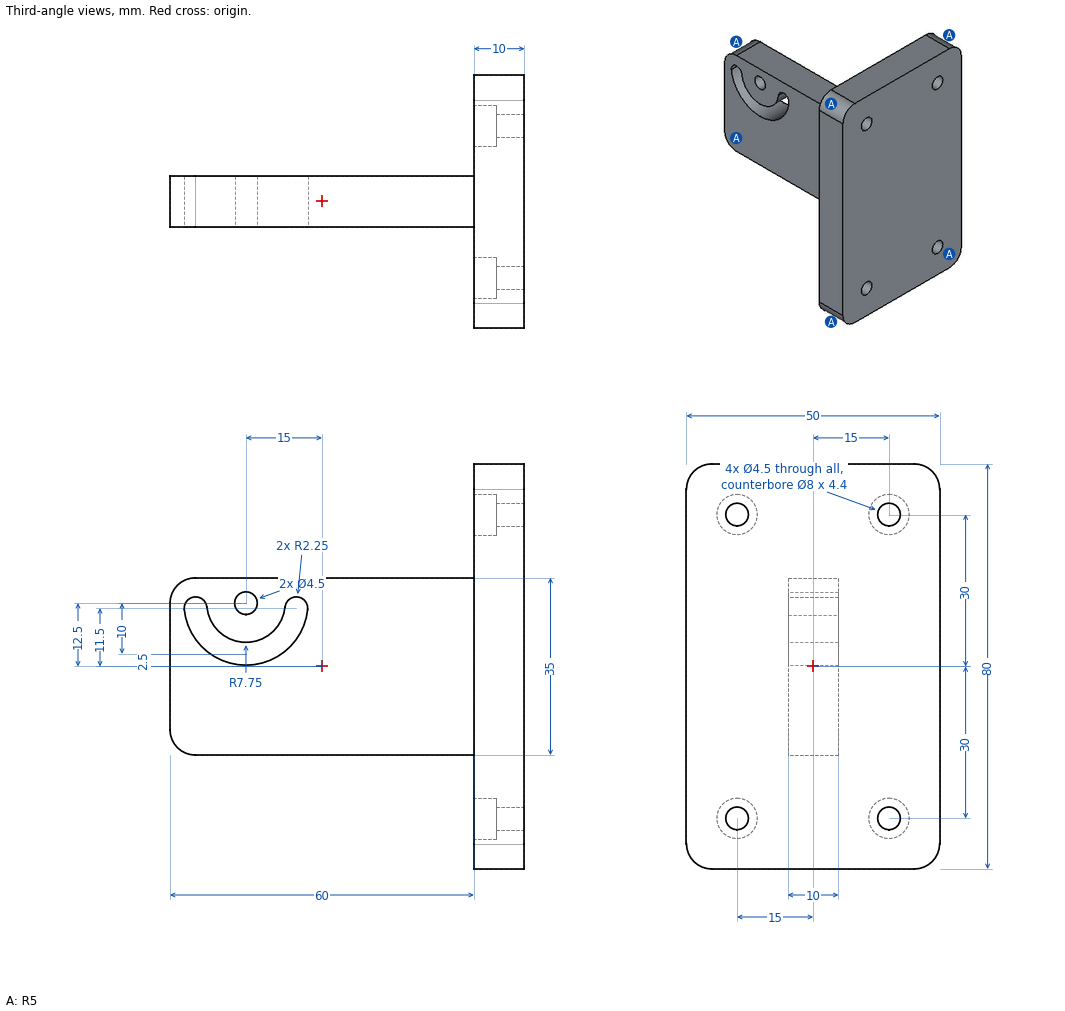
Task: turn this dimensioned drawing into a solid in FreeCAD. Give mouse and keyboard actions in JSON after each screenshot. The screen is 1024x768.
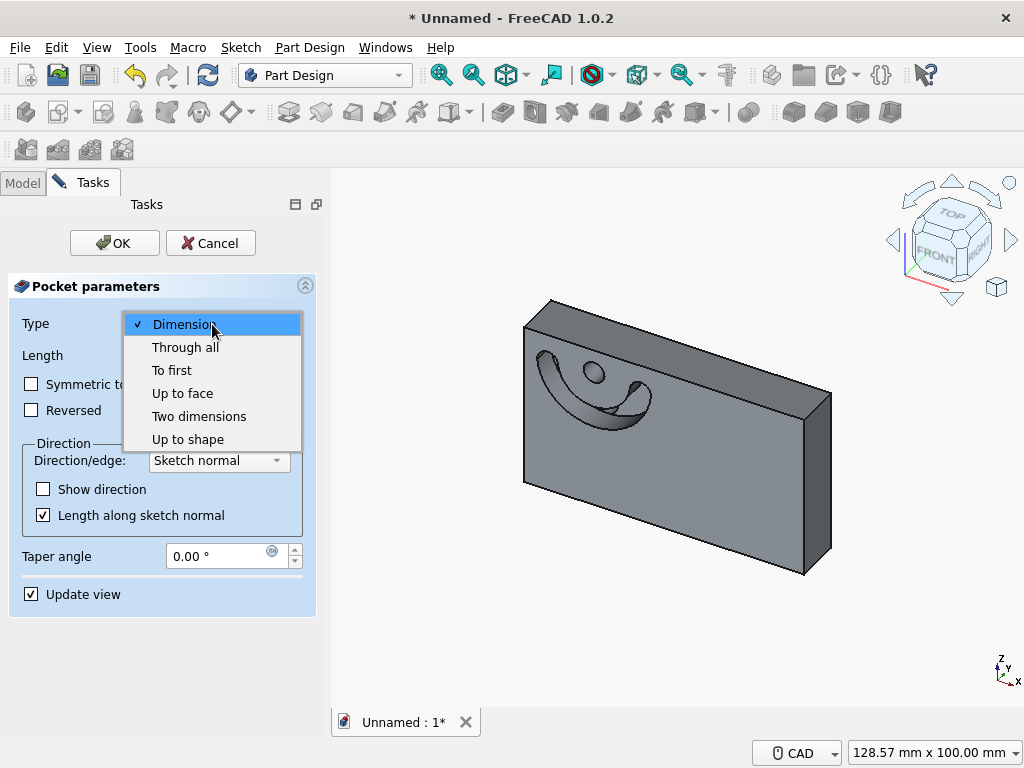
{"action": "left_click", "coordinate": [212, 348]}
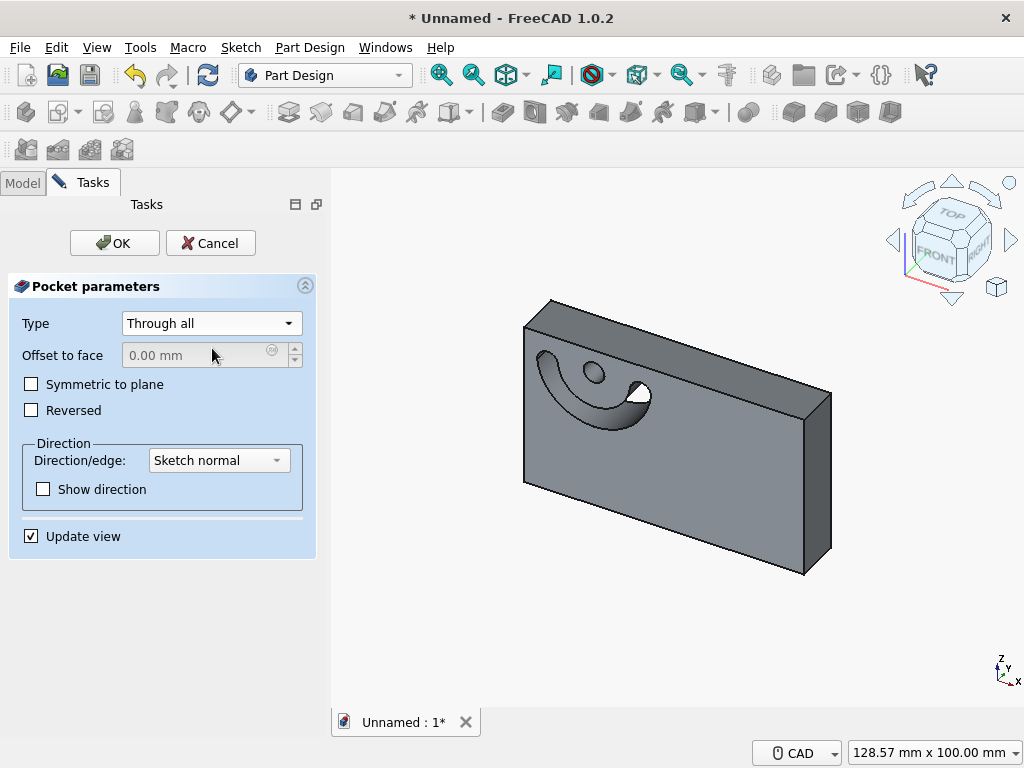
{"action": "left_click", "coordinate": [115, 243]}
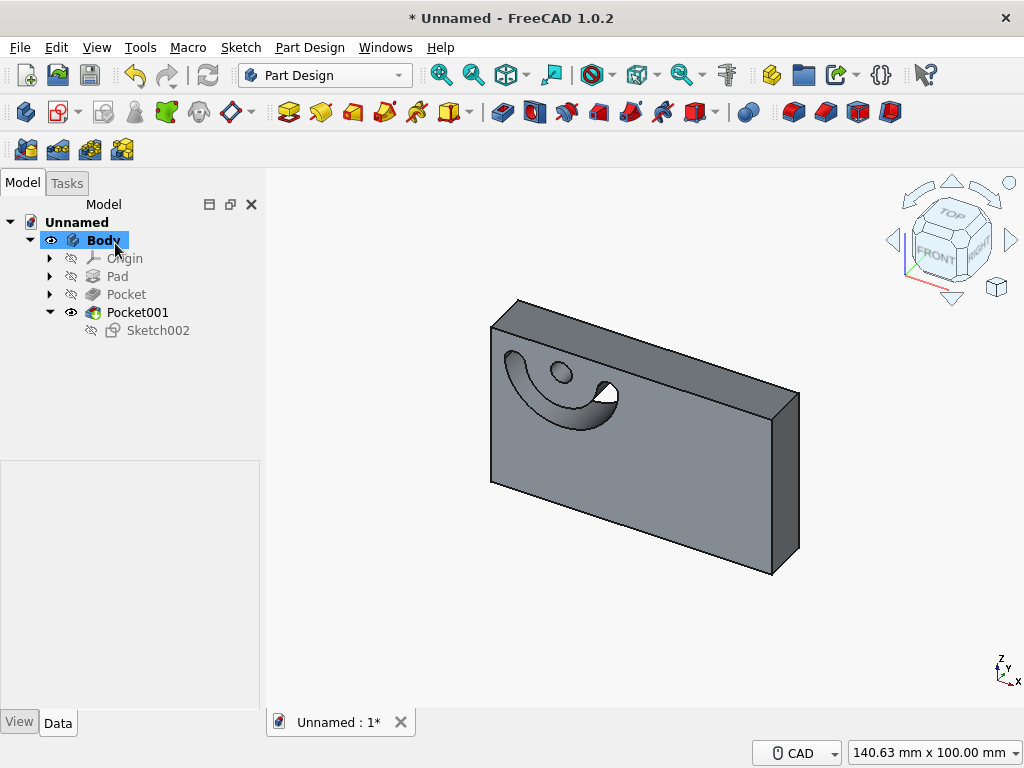
{"action": "left_click", "coordinate": [785, 439]}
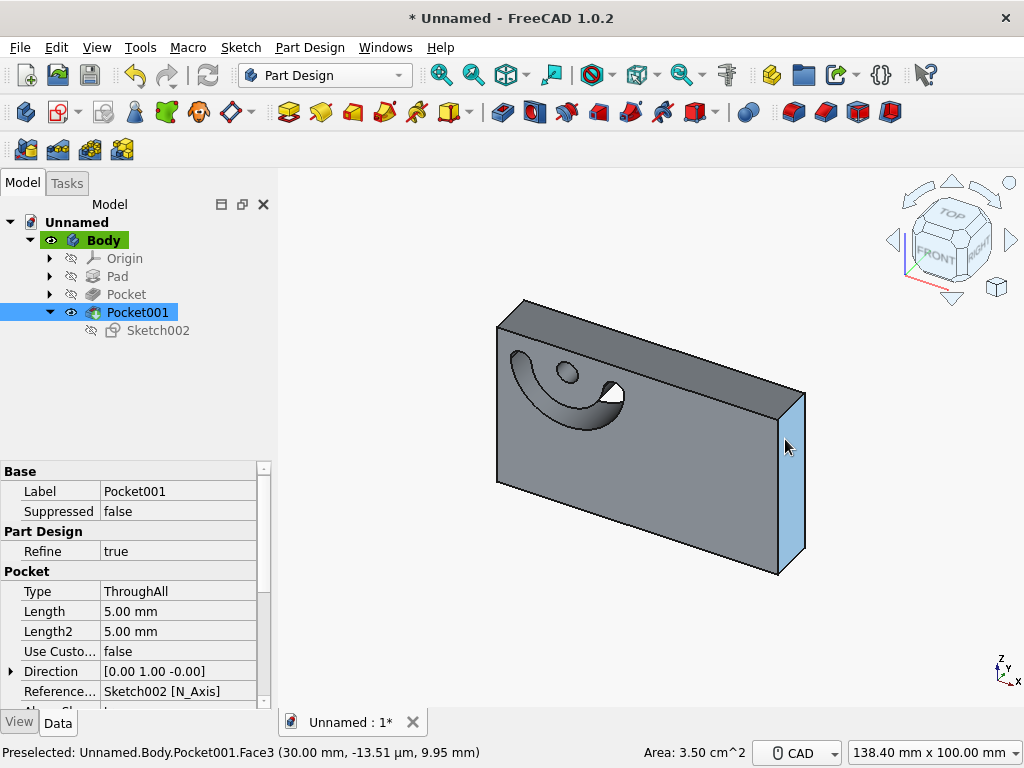
{"action": "left_click", "coordinate": [58, 112]}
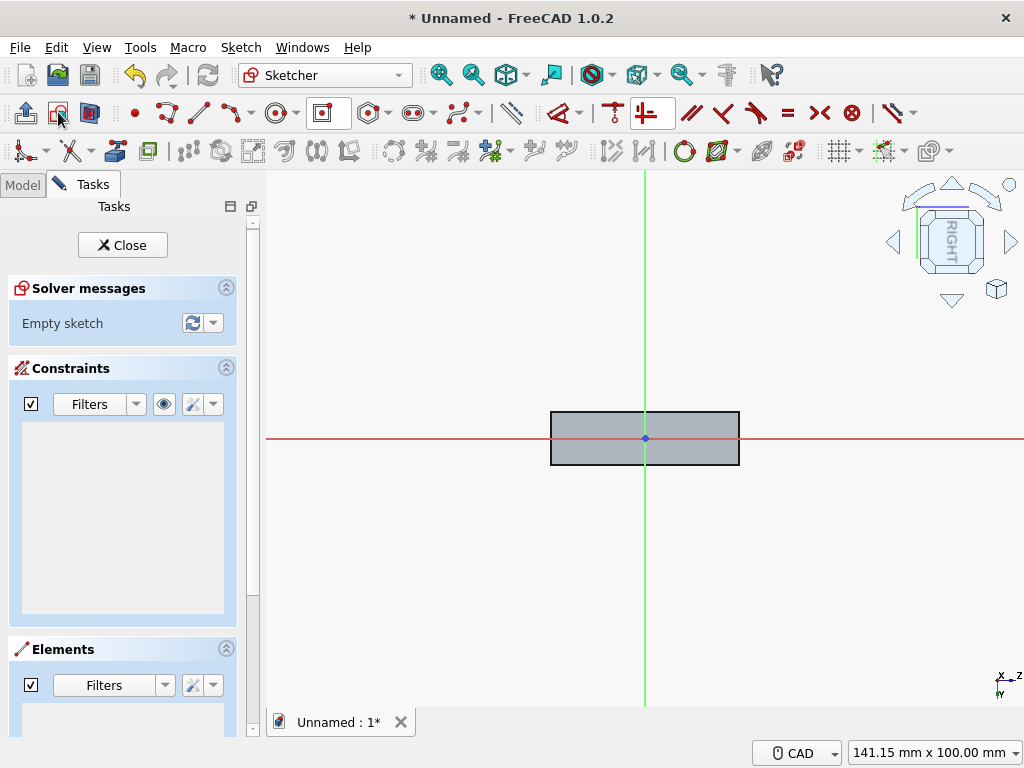
{"action": "scroll", "coordinate": [294, 439], "scroll_direction": "down", "scroll_amount": 1}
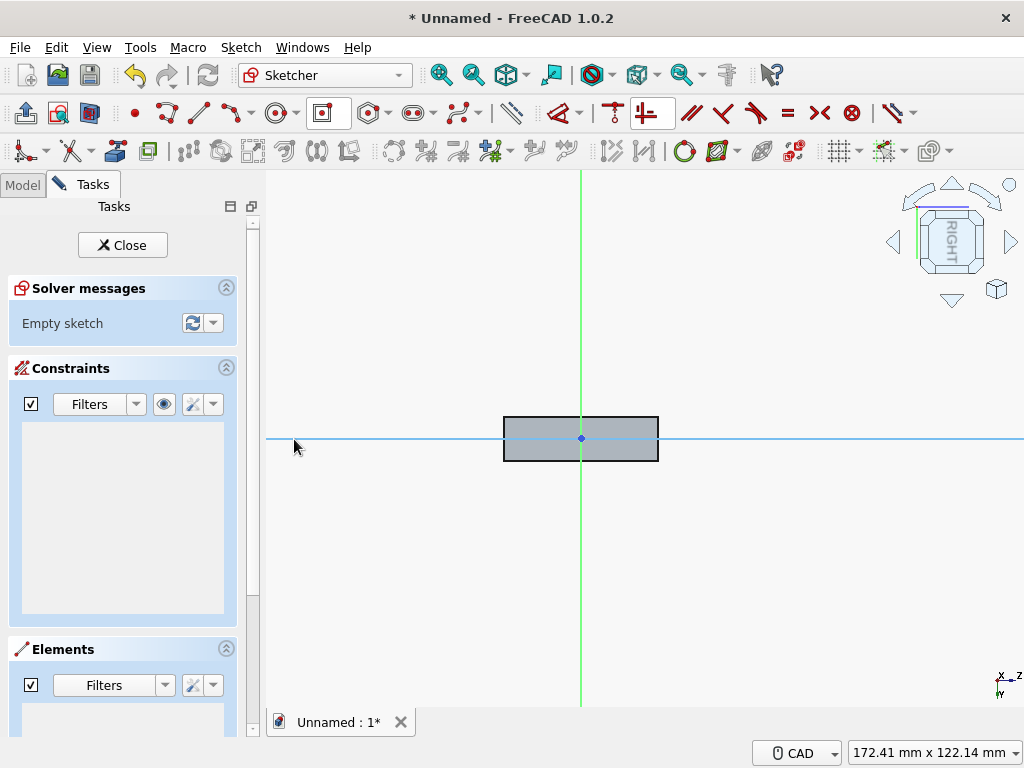
{"action": "left_click", "coordinate": [322, 114]}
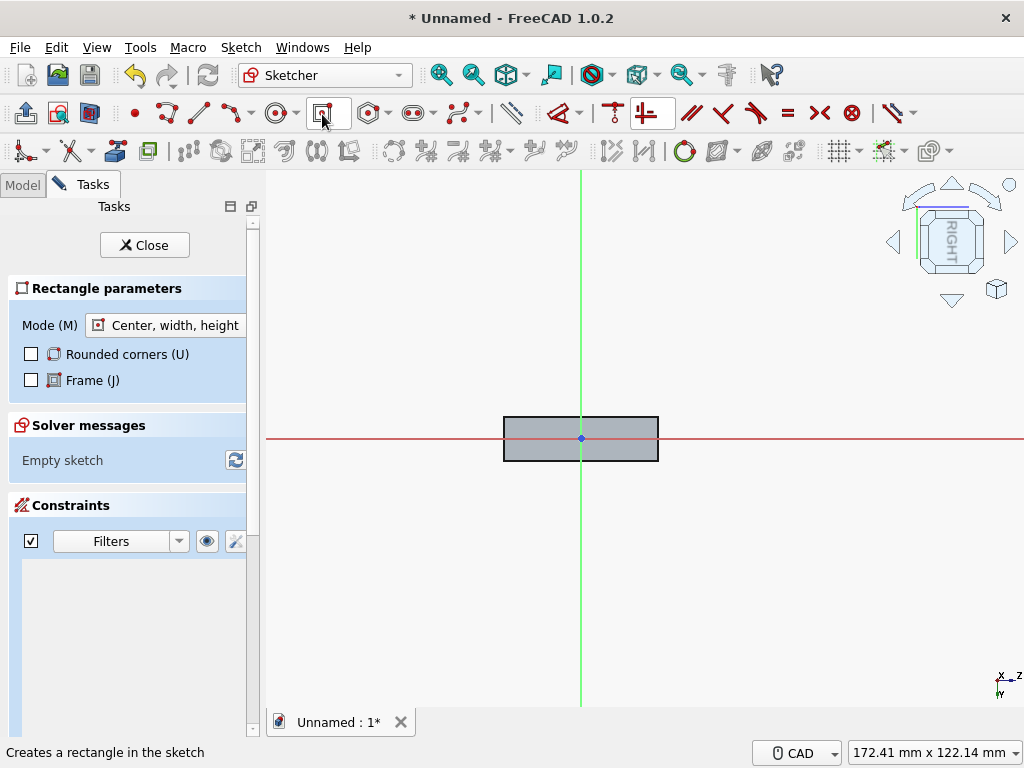
{"action": "left_click", "coordinate": [581, 439]}
{"action": "left_click", "coordinate": [757, 329]}
{"action": "key", "text": "Escape"}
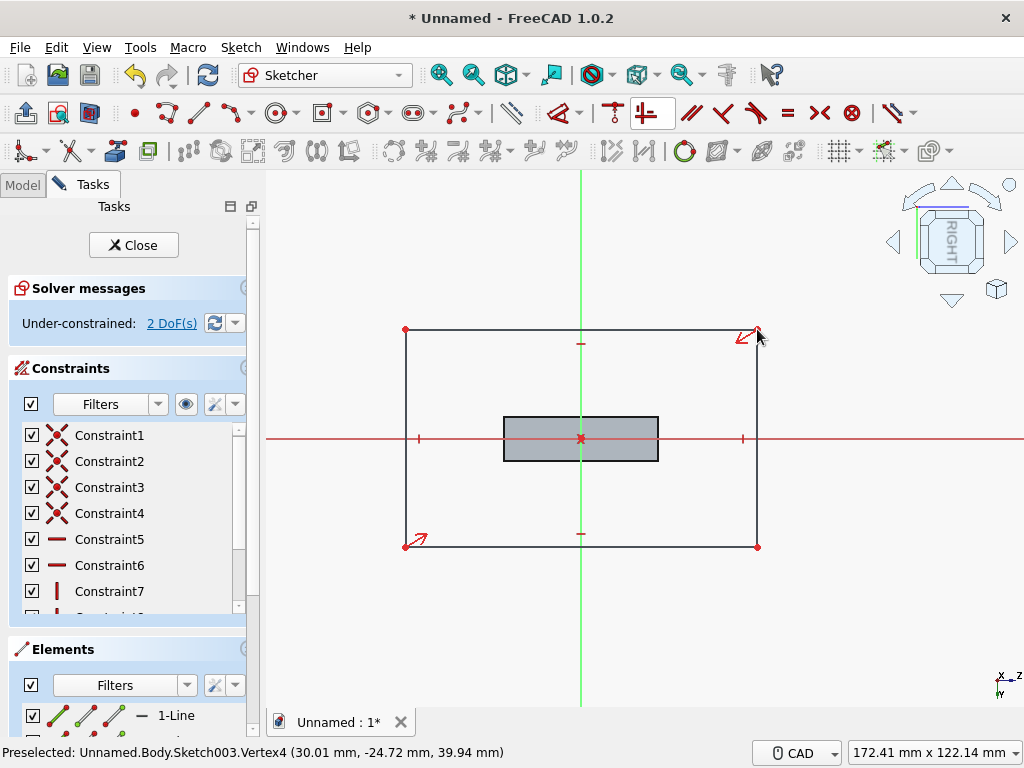
{"action": "left_click", "coordinate": [558, 114]}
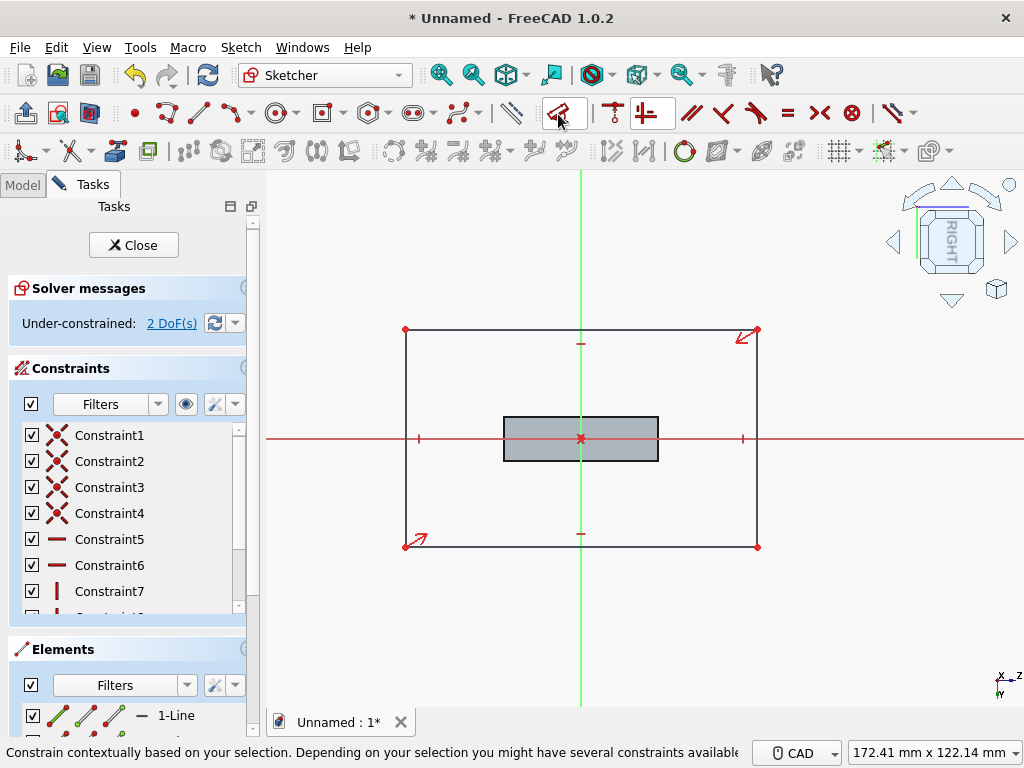
{"action": "left_click", "coordinate": [511, 547]}
{"action": "left_click", "coordinate": [501, 581]}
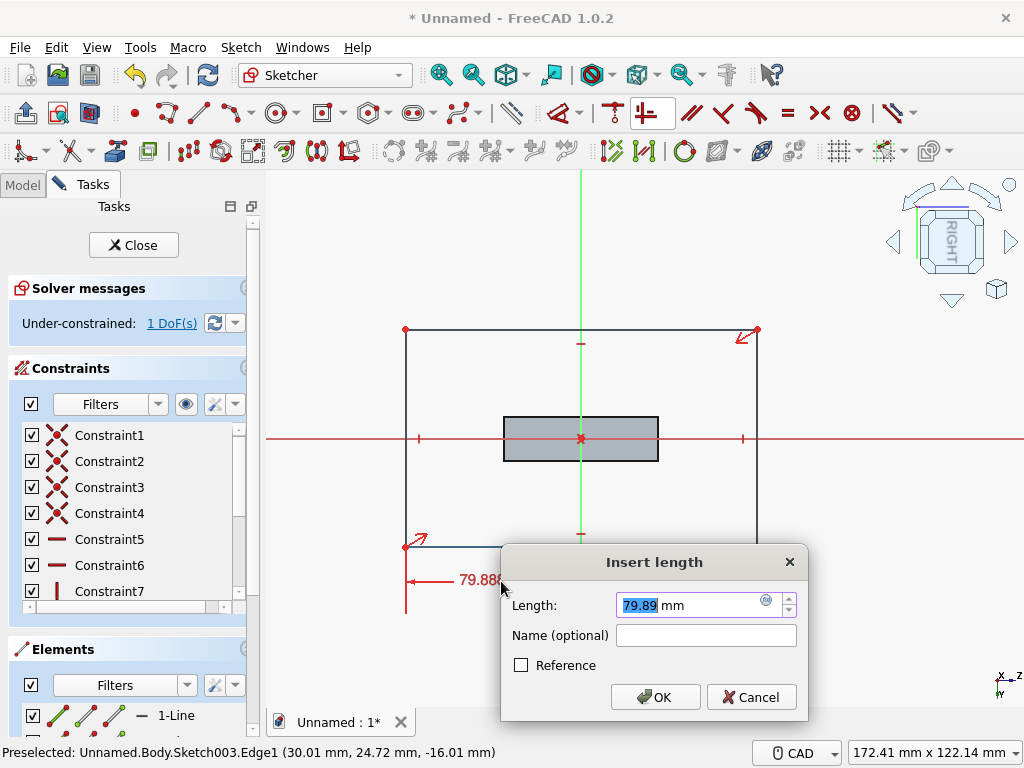
{"action": "type", "text": "80"}
{"action": "key", "text": "Return"}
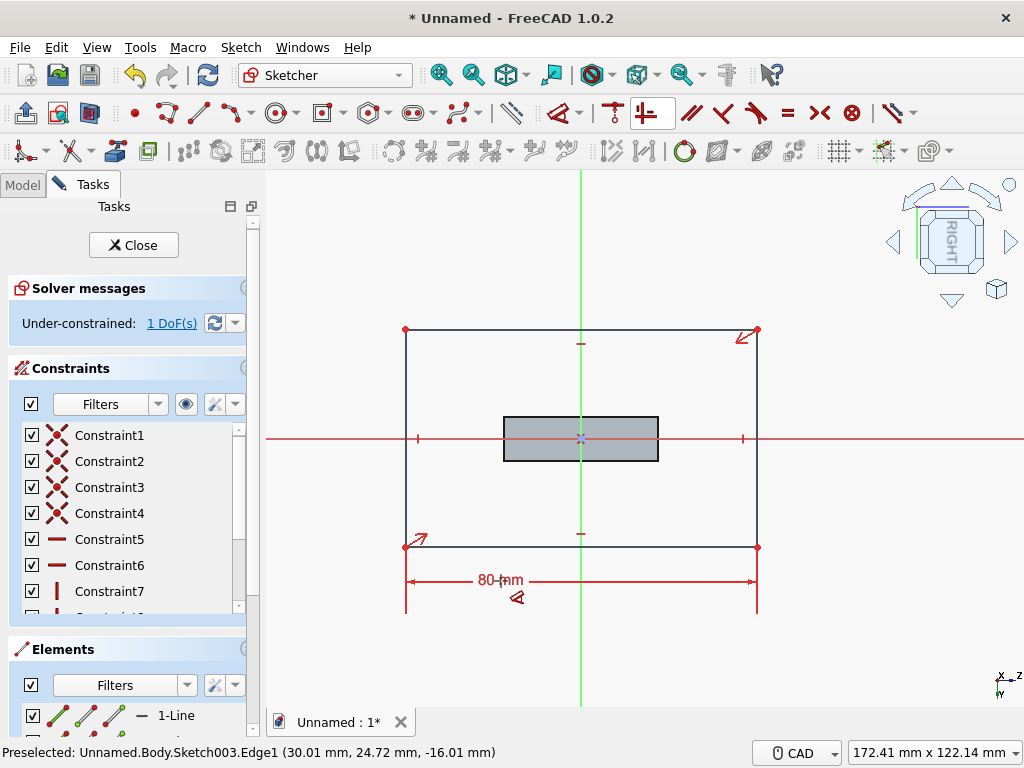
{"action": "left_click", "coordinate": [757, 482]}
{"action": "left_click", "coordinate": [791, 389]}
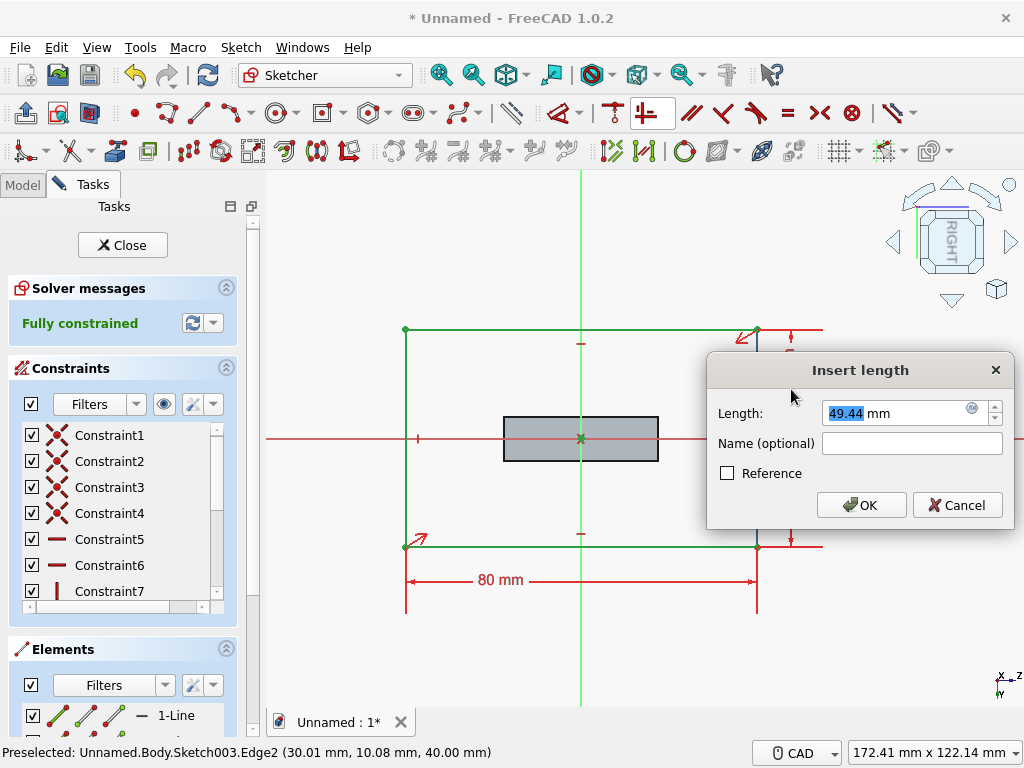
{"action": "type", "text": "50"}
{"action": "key", "text": "Return"}
{"action": "key", "text": "Escape"}